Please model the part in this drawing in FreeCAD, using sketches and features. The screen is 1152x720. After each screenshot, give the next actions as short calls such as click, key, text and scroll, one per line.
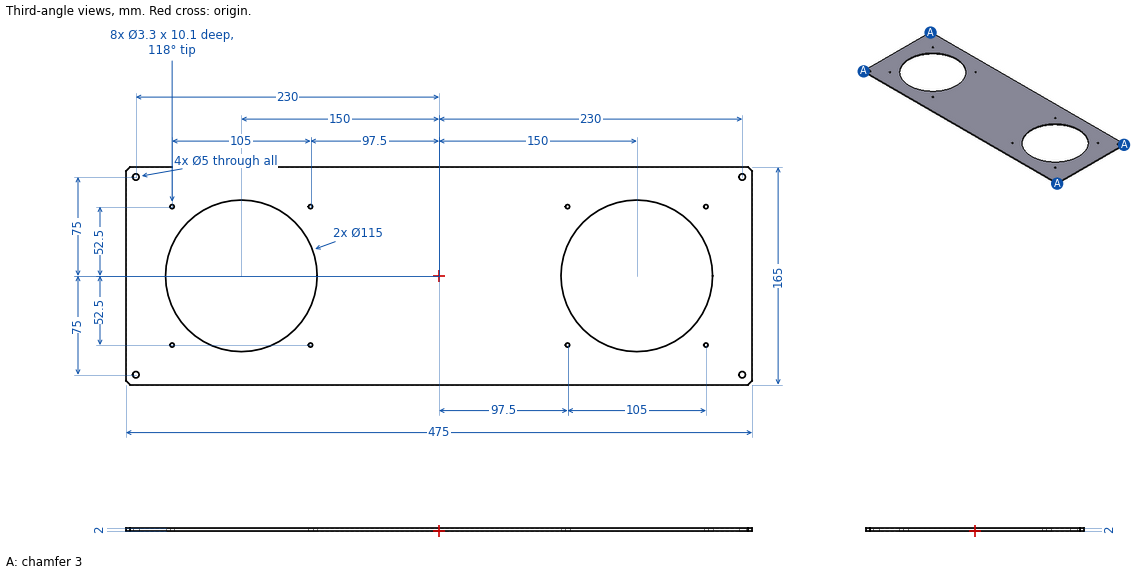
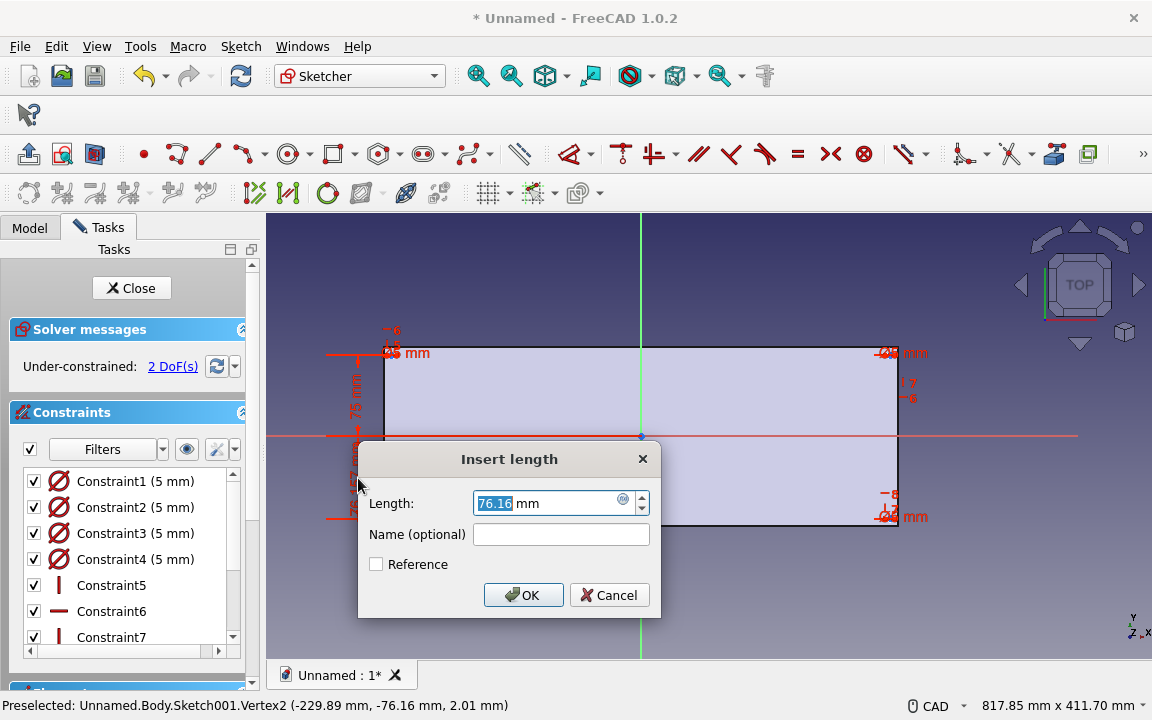
text(75)
key(Return)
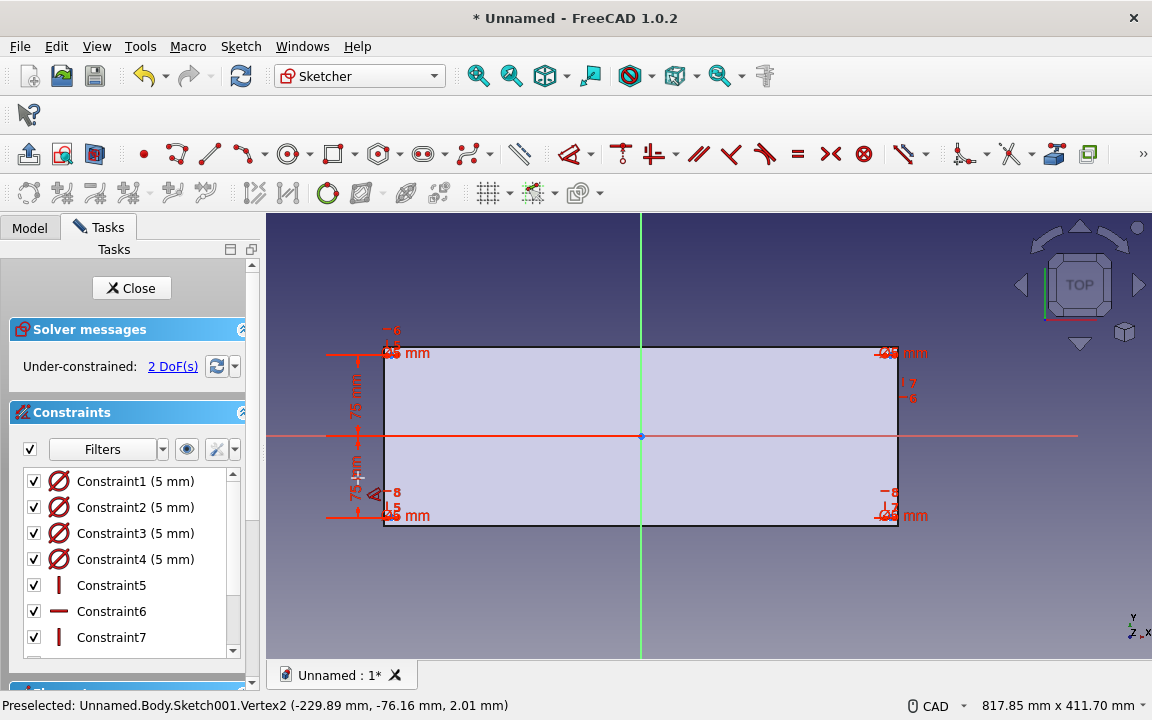
click(392, 355)
click(517, 321)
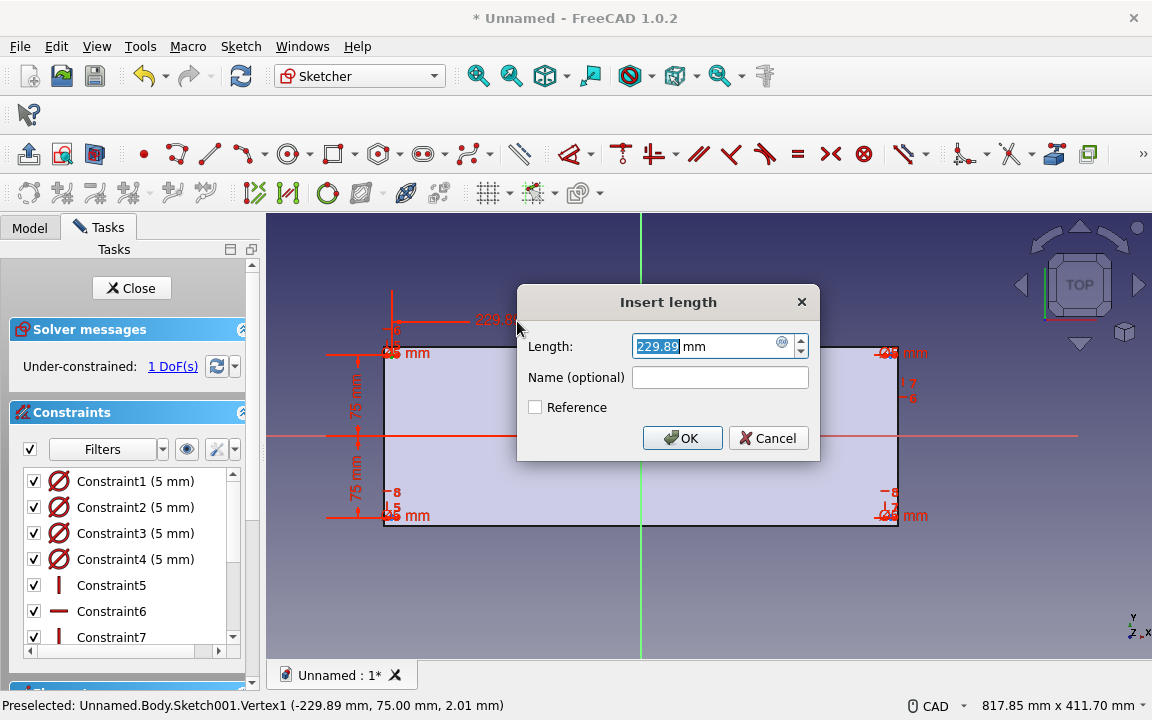
text(230)
key(Return)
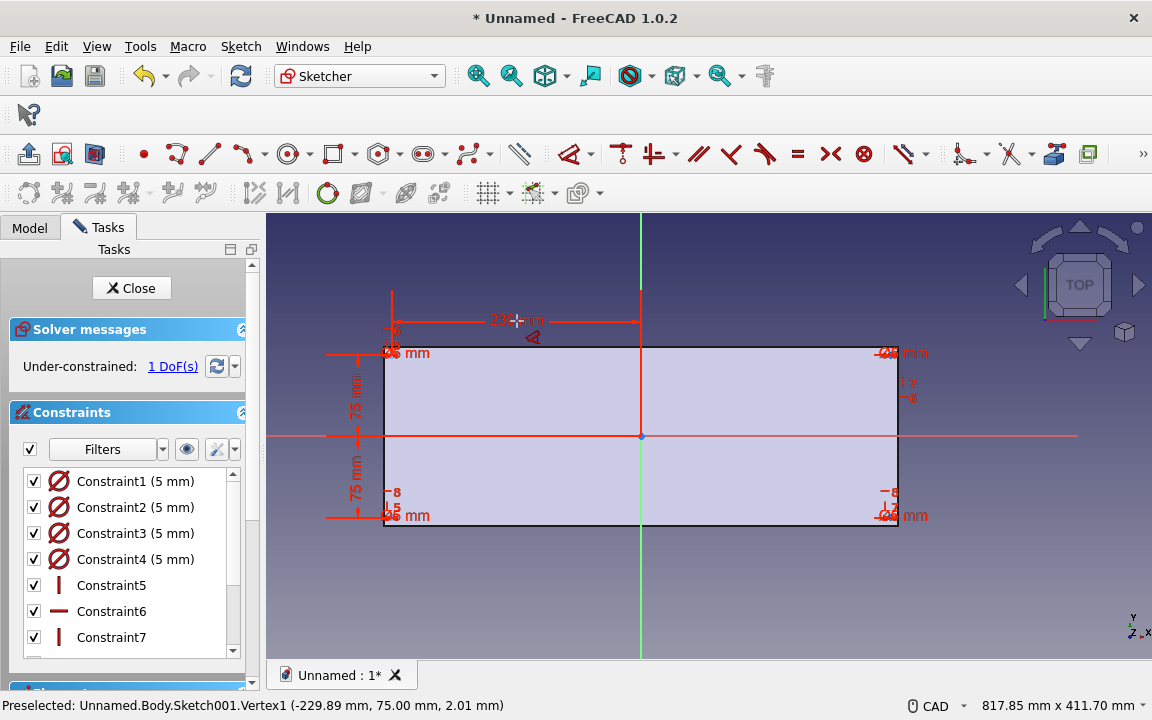
click(890, 355)
click(766, 321)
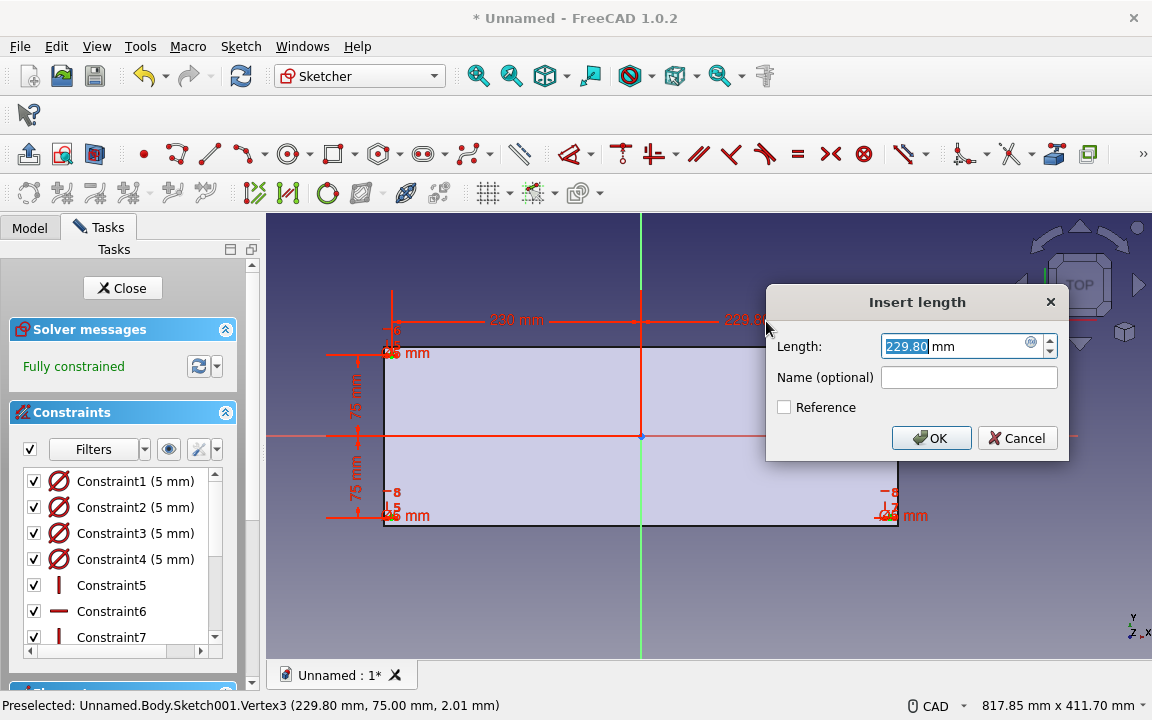
text(230)
key(Return)
key(Escape)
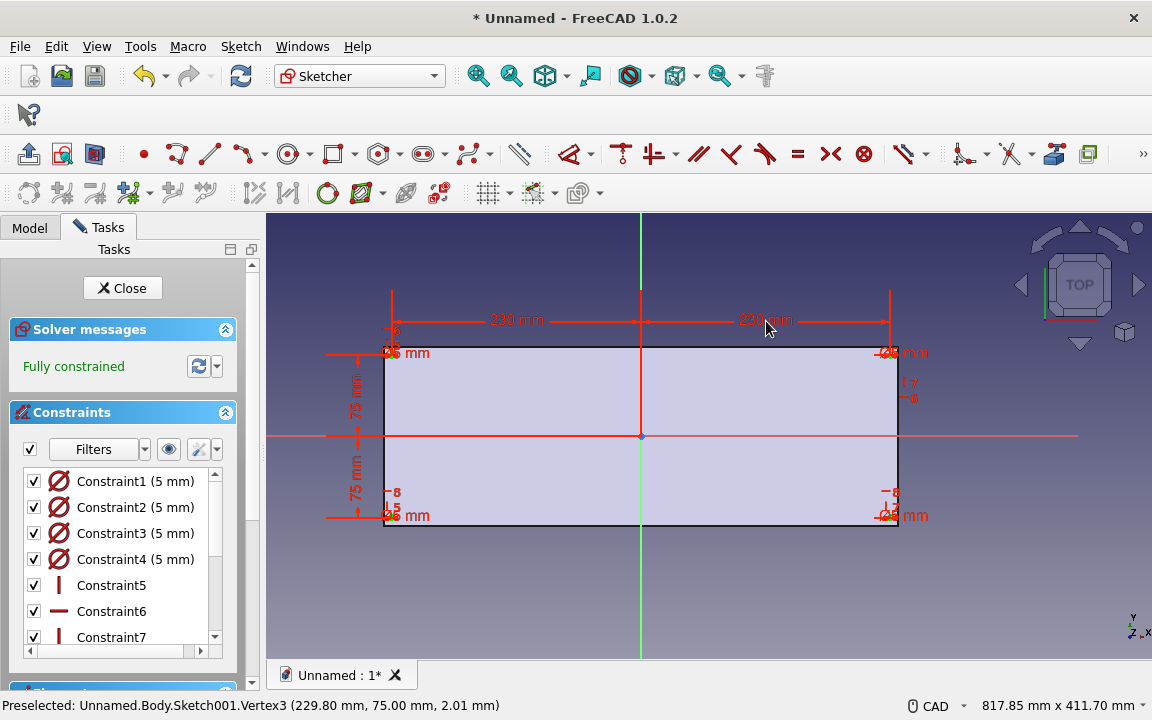
click(123, 288)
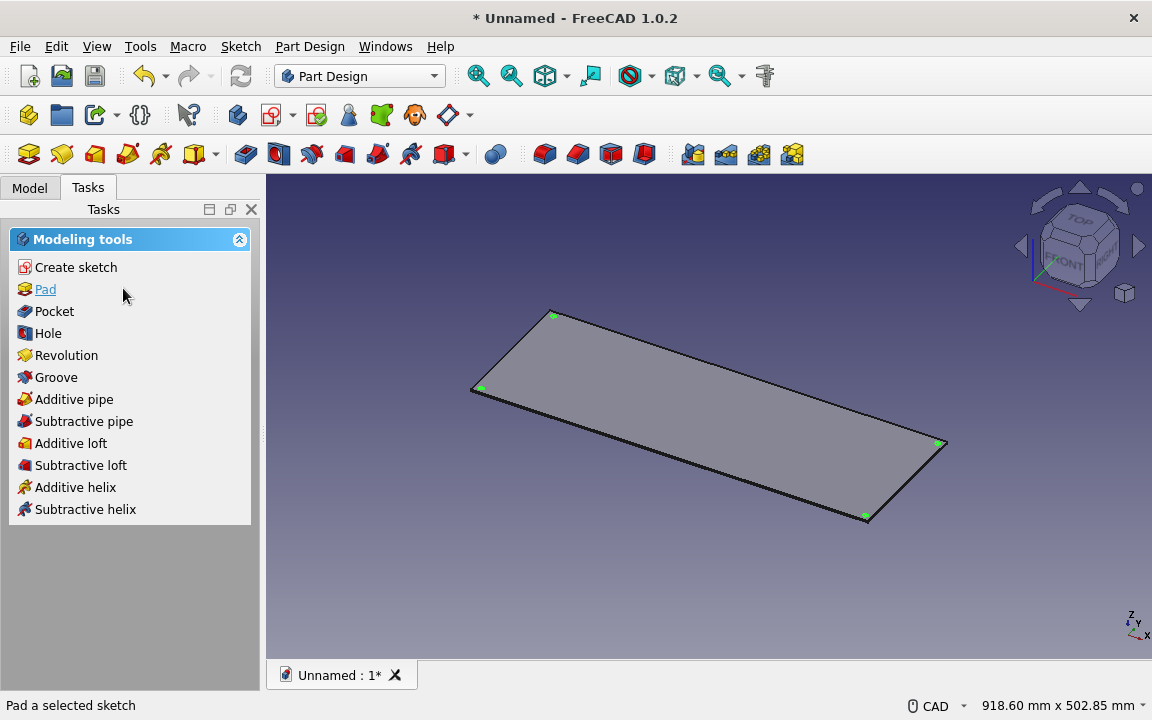
click(279, 154)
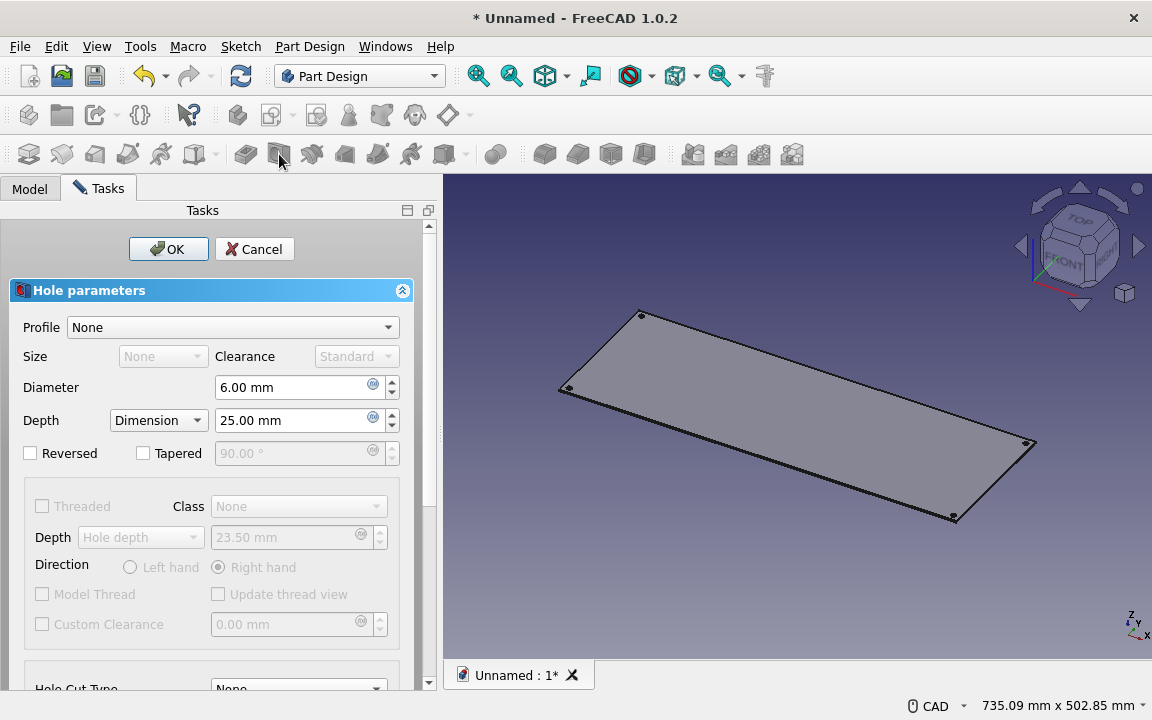
triple_click(300, 388)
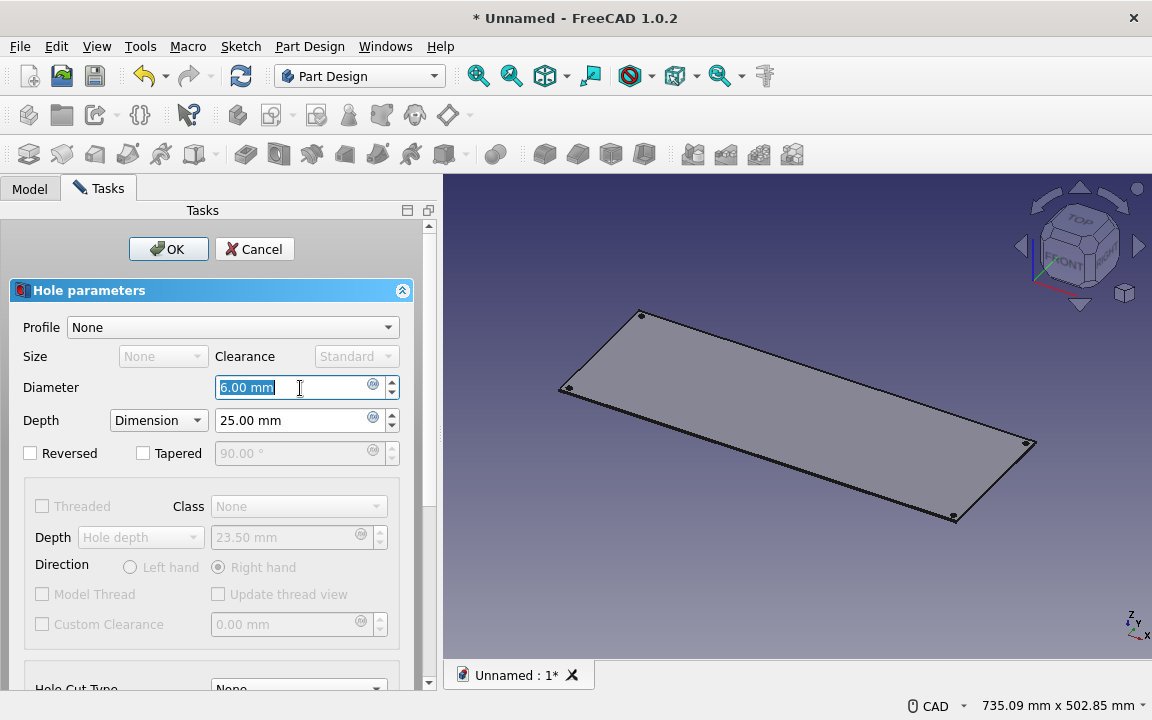
text(5)
key(Tab)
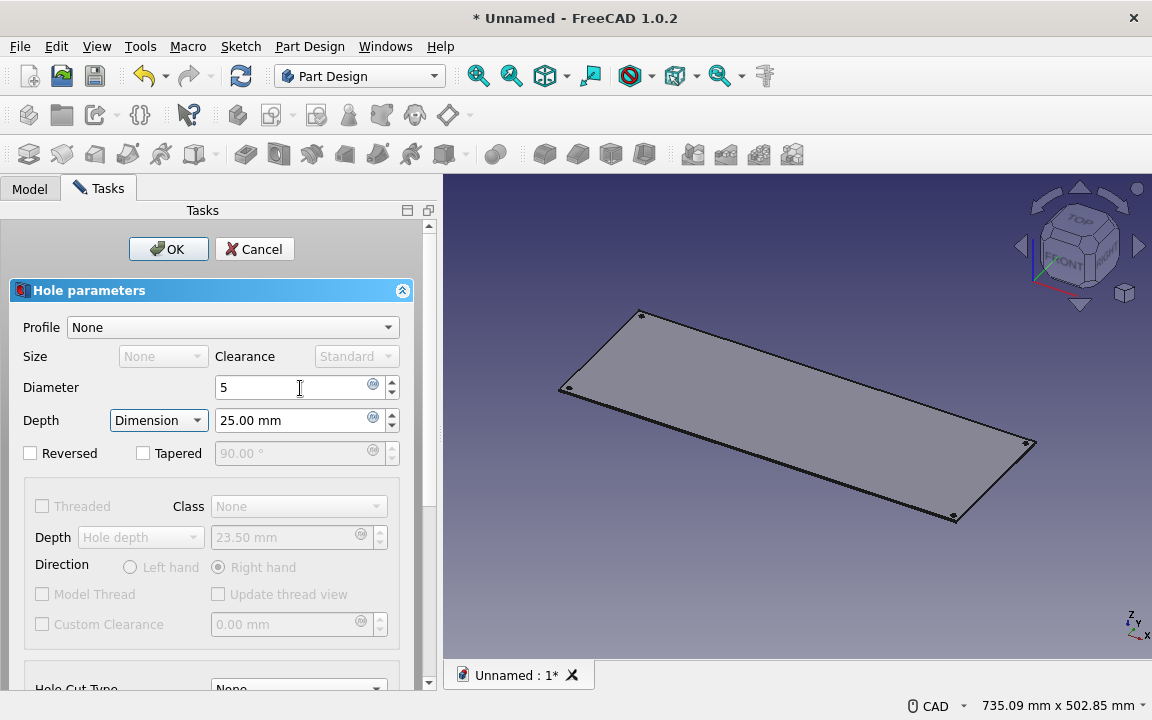
click(160, 420)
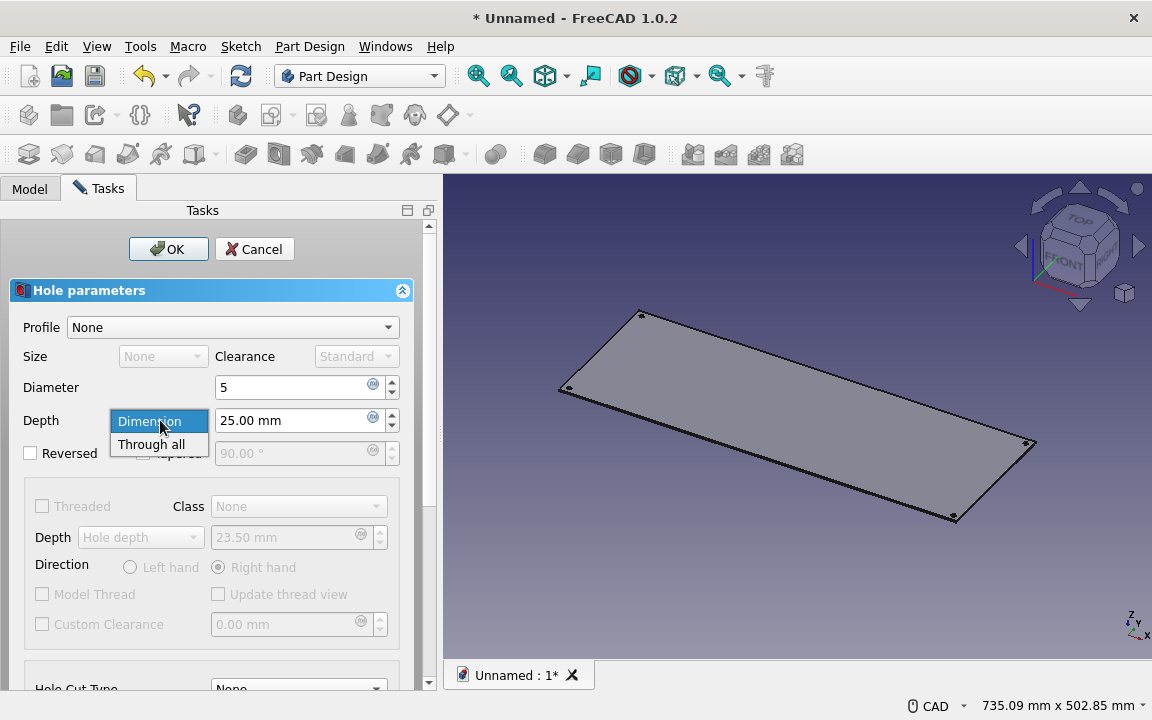
click(158, 444)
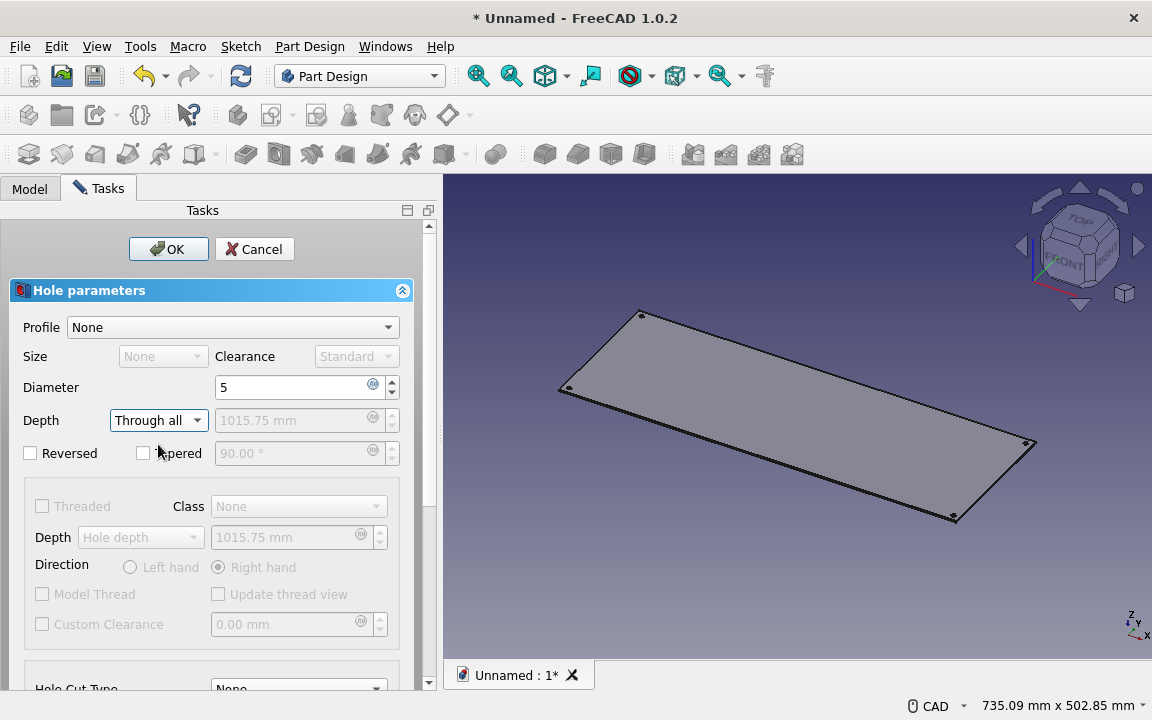
click(169, 249)